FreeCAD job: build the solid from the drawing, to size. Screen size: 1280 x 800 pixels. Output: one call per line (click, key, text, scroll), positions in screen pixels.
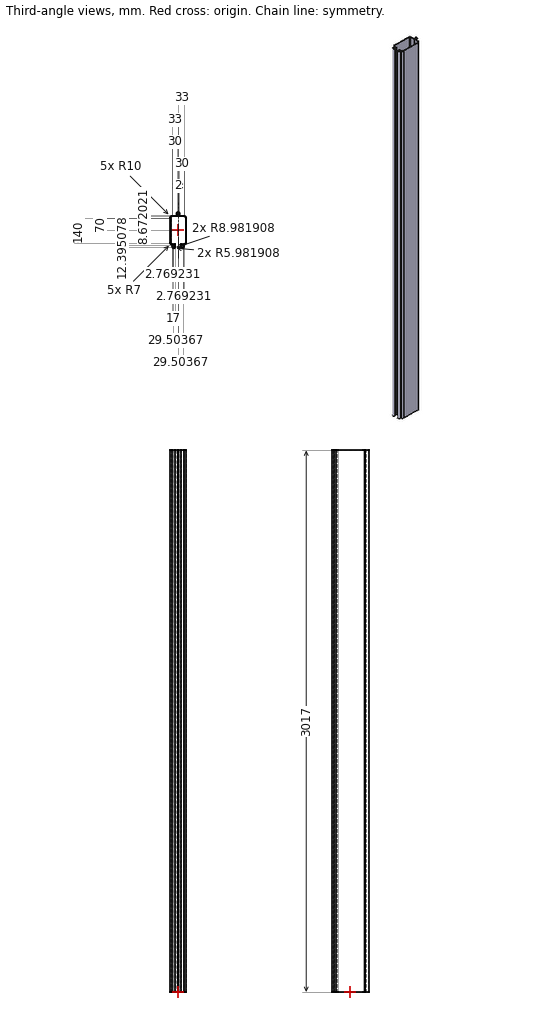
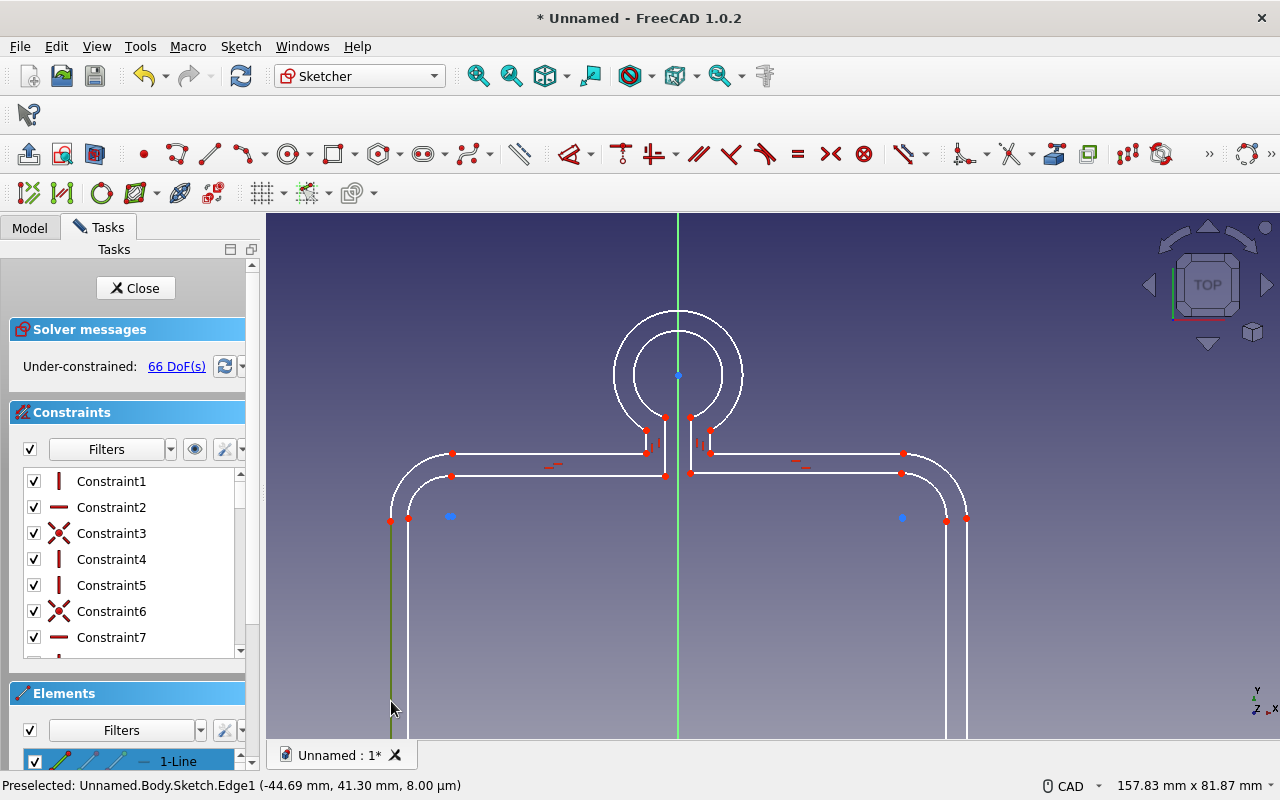
scroll(713, 316, down, 7)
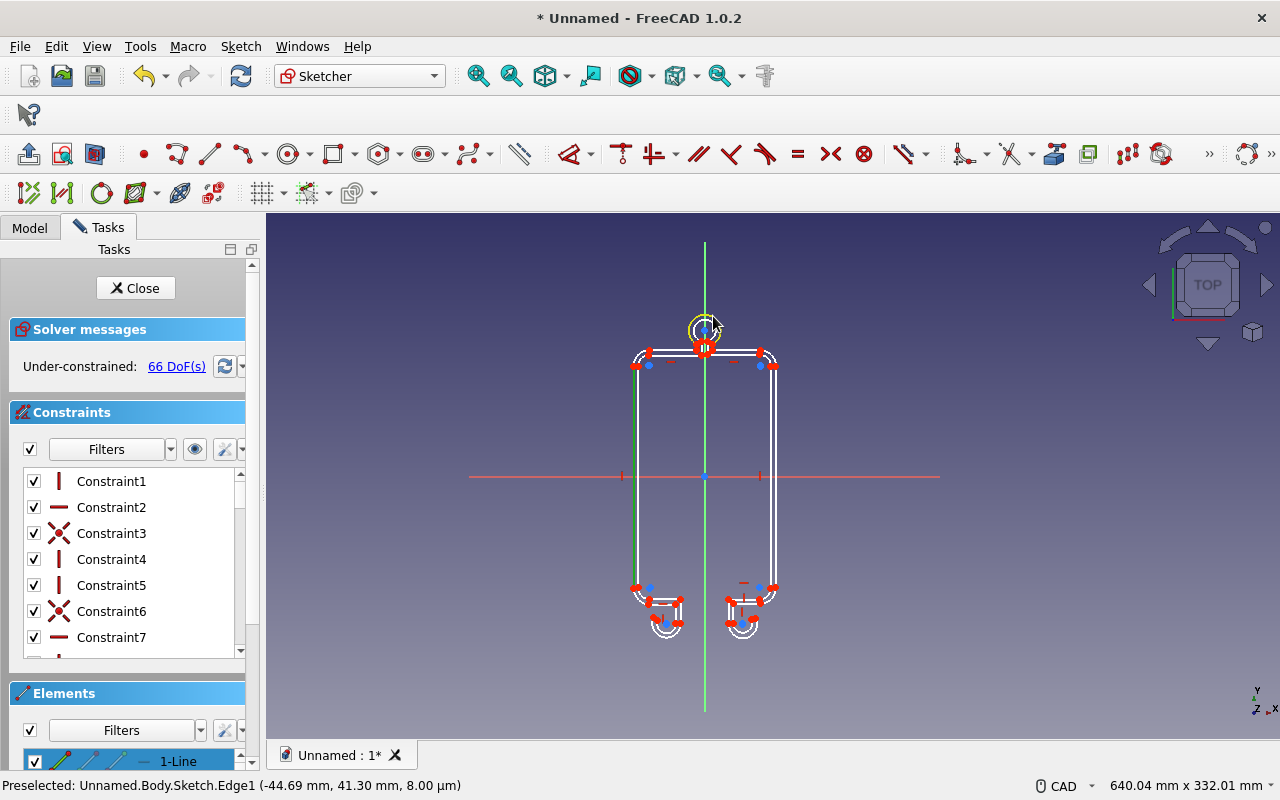
scroll(636, 596, up, 6)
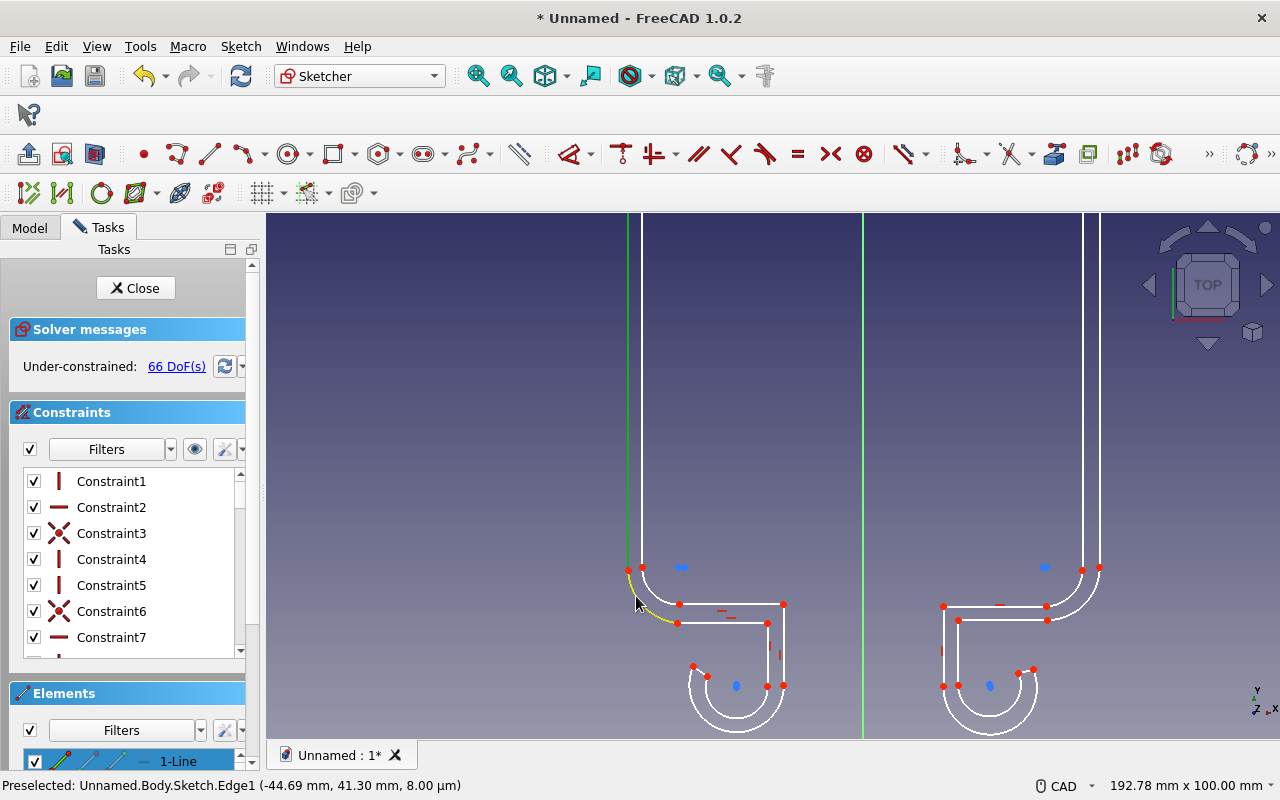
click(634, 593)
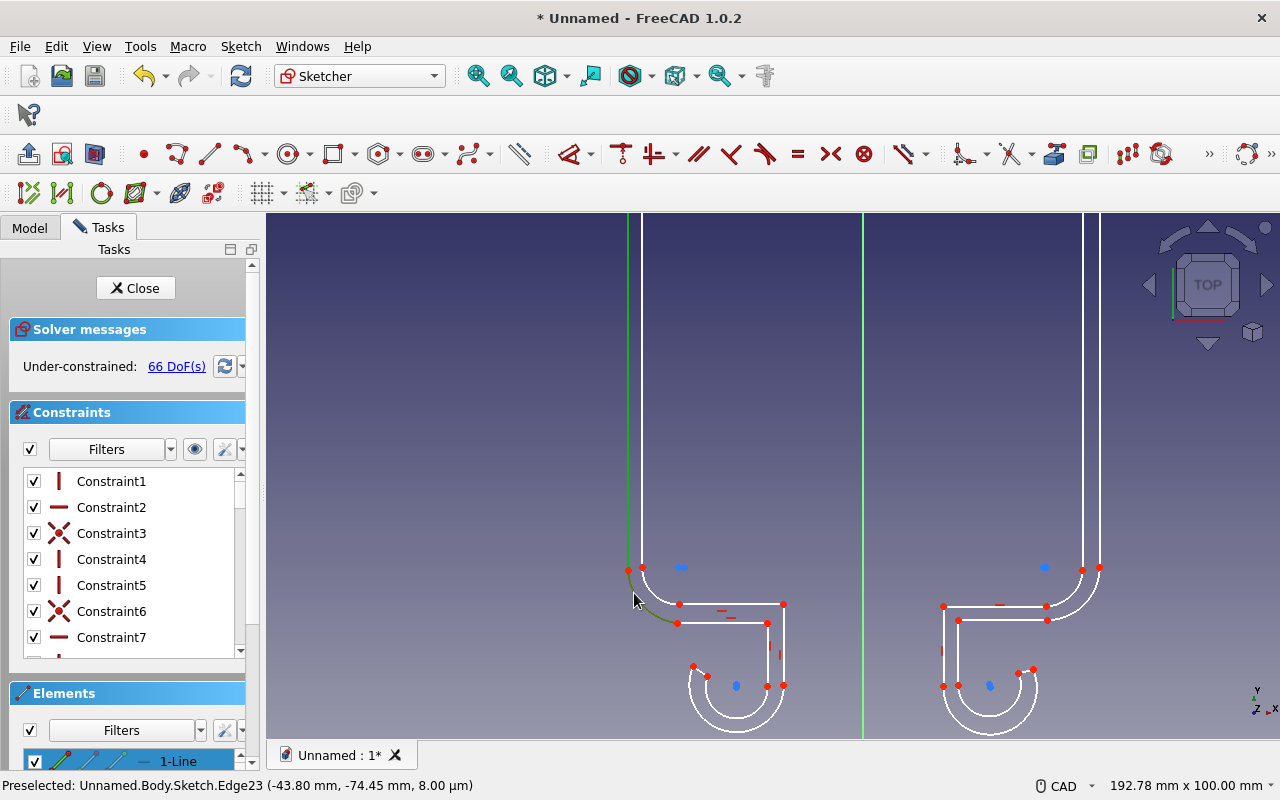
click(765, 154)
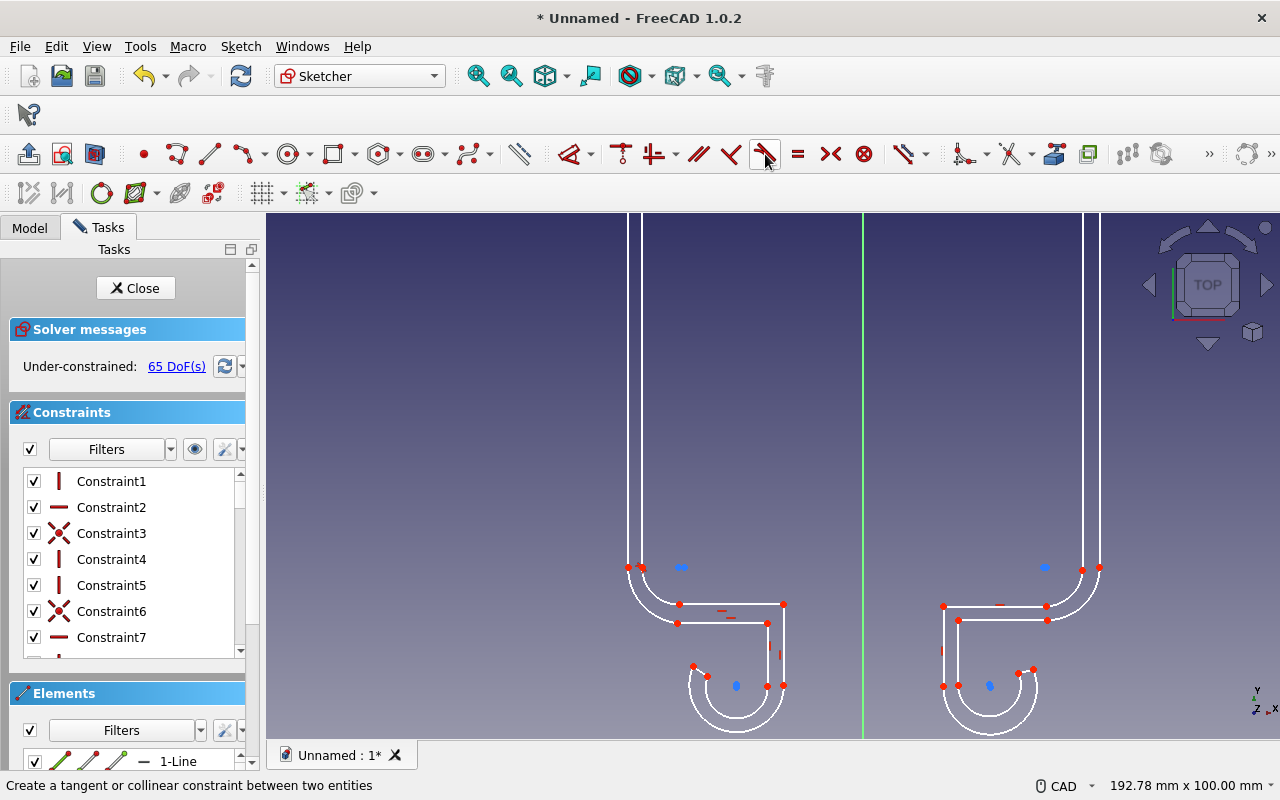
click(628, 347)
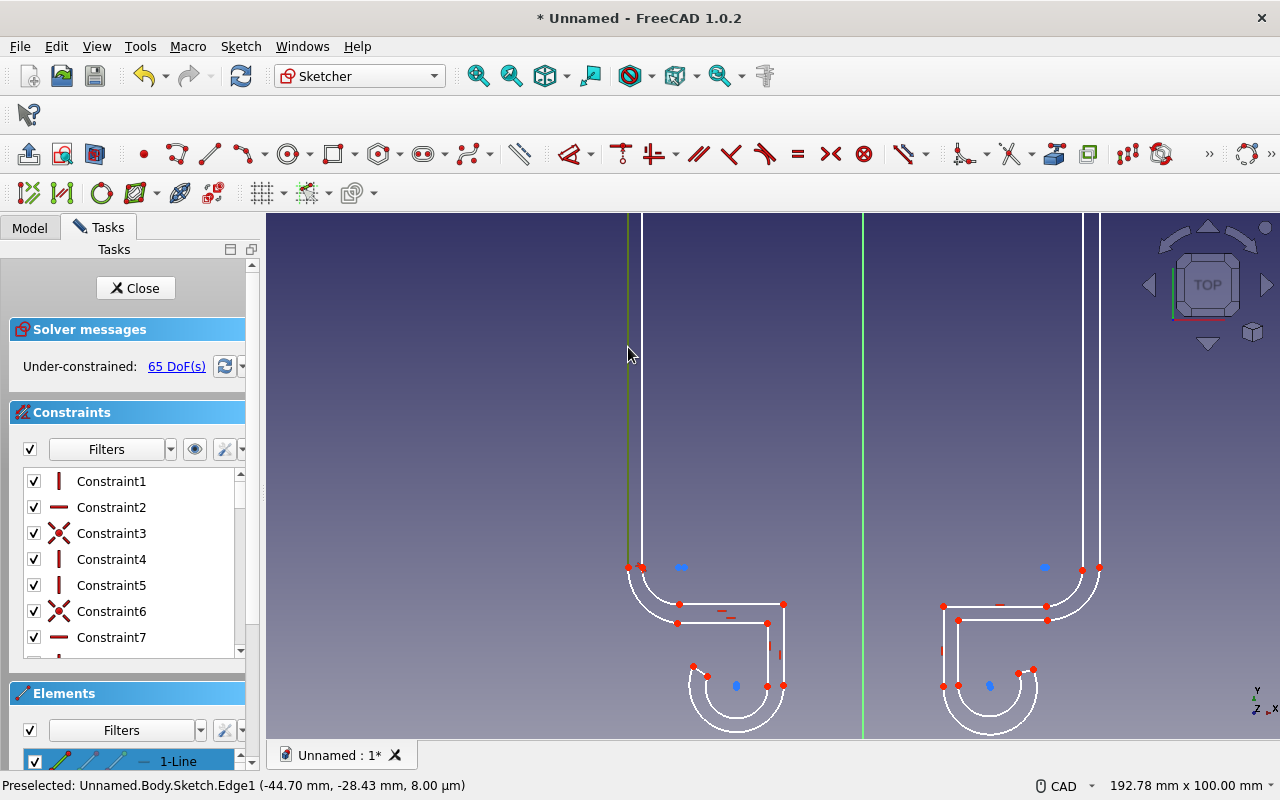
scroll(636, 597, down, 6)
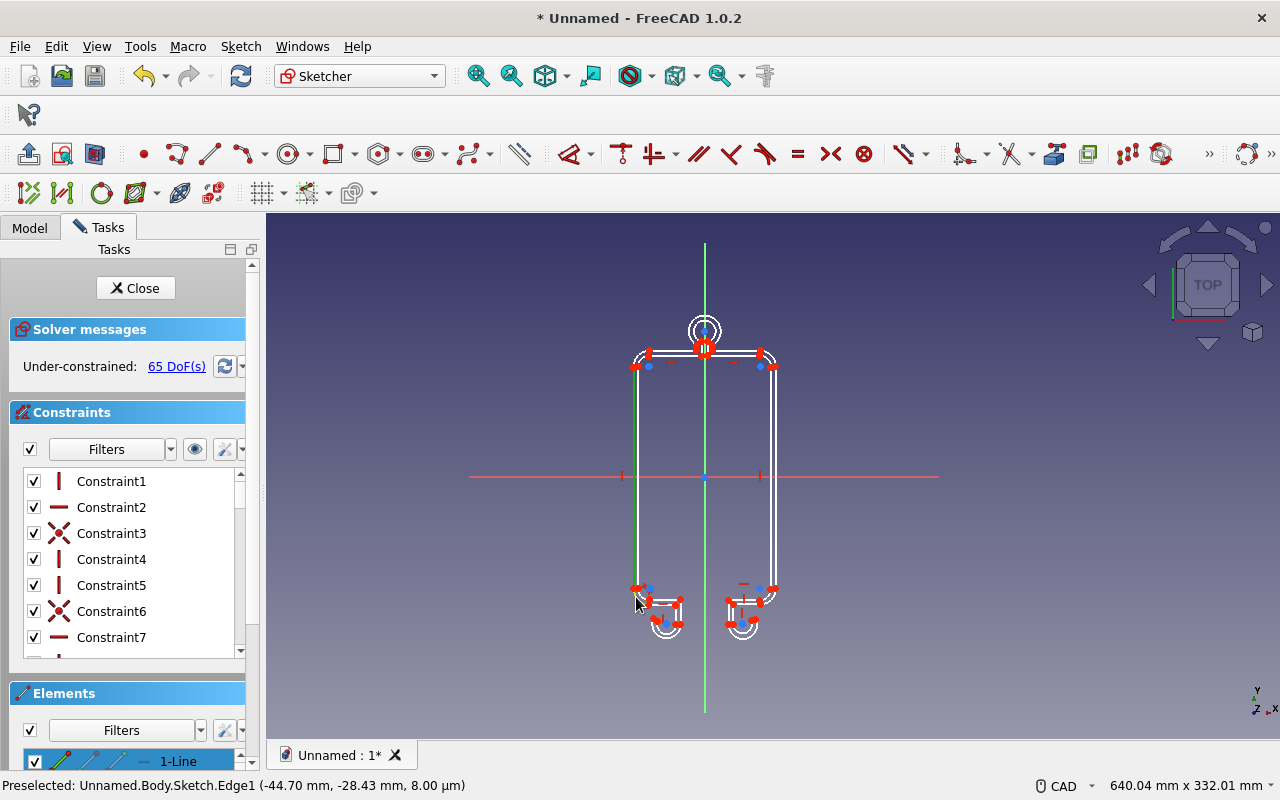
scroll(642, 353, up, 6)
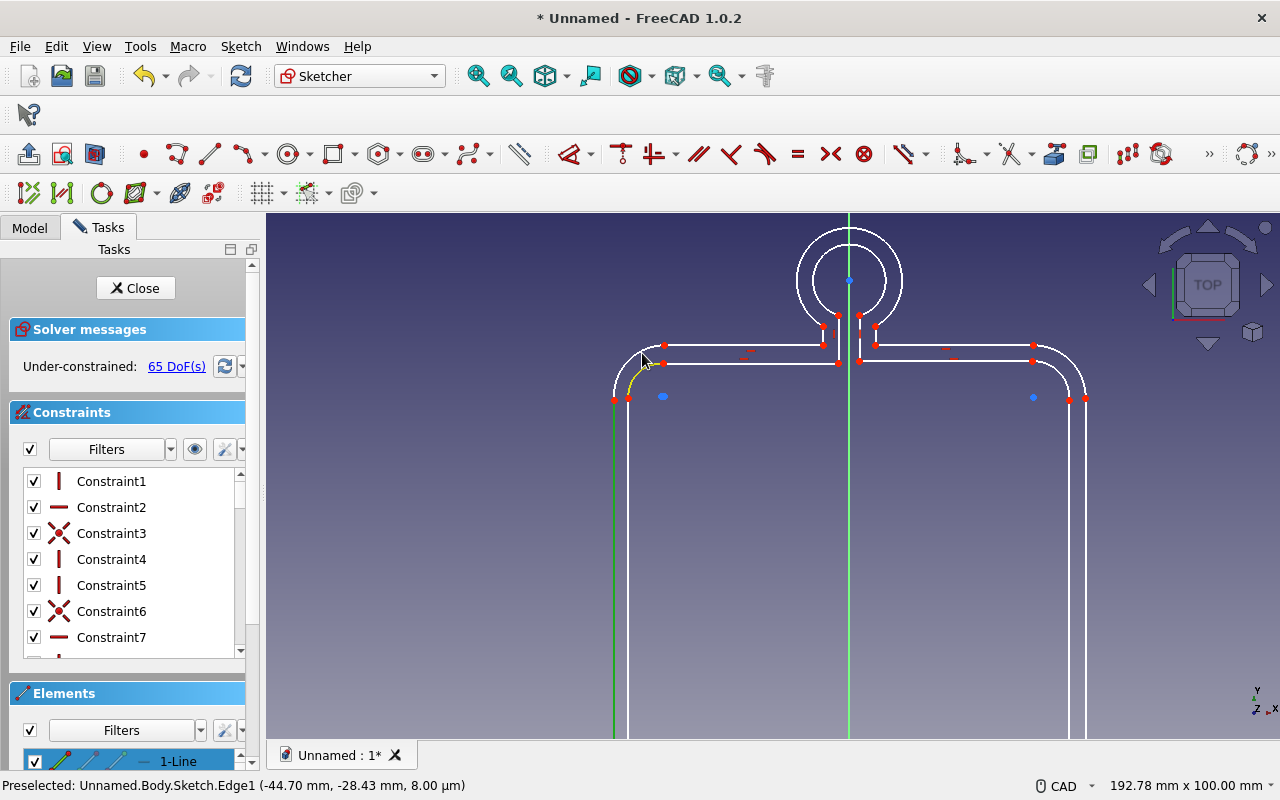
click(641, 351)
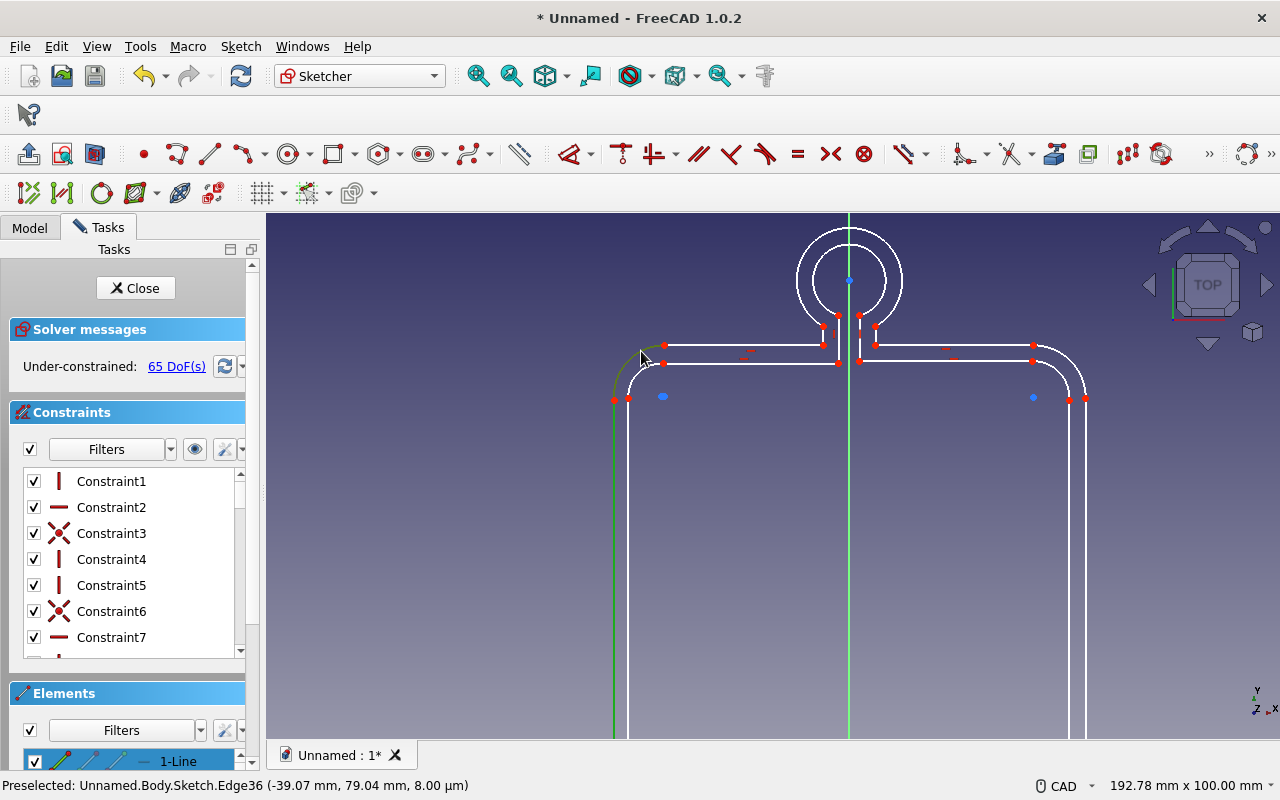
click(765, 154)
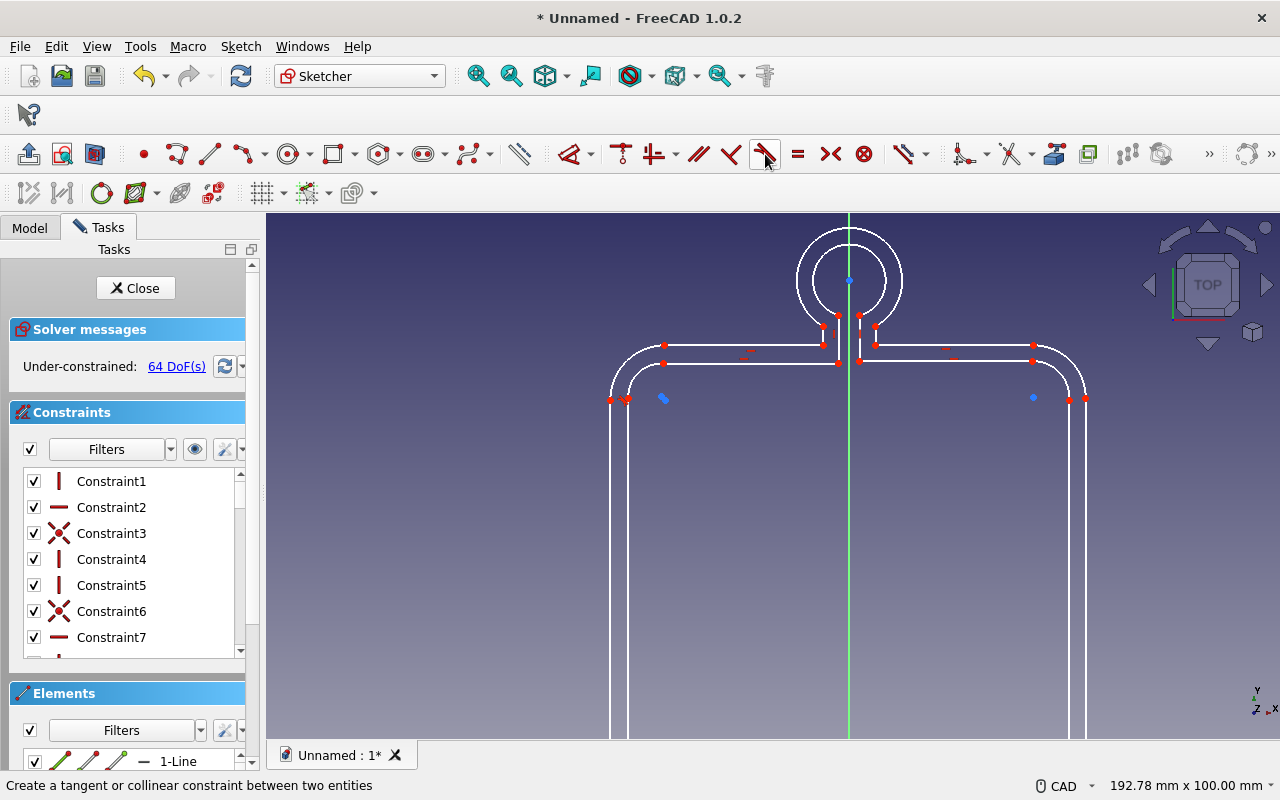
scroll(642, 353, down, 6)